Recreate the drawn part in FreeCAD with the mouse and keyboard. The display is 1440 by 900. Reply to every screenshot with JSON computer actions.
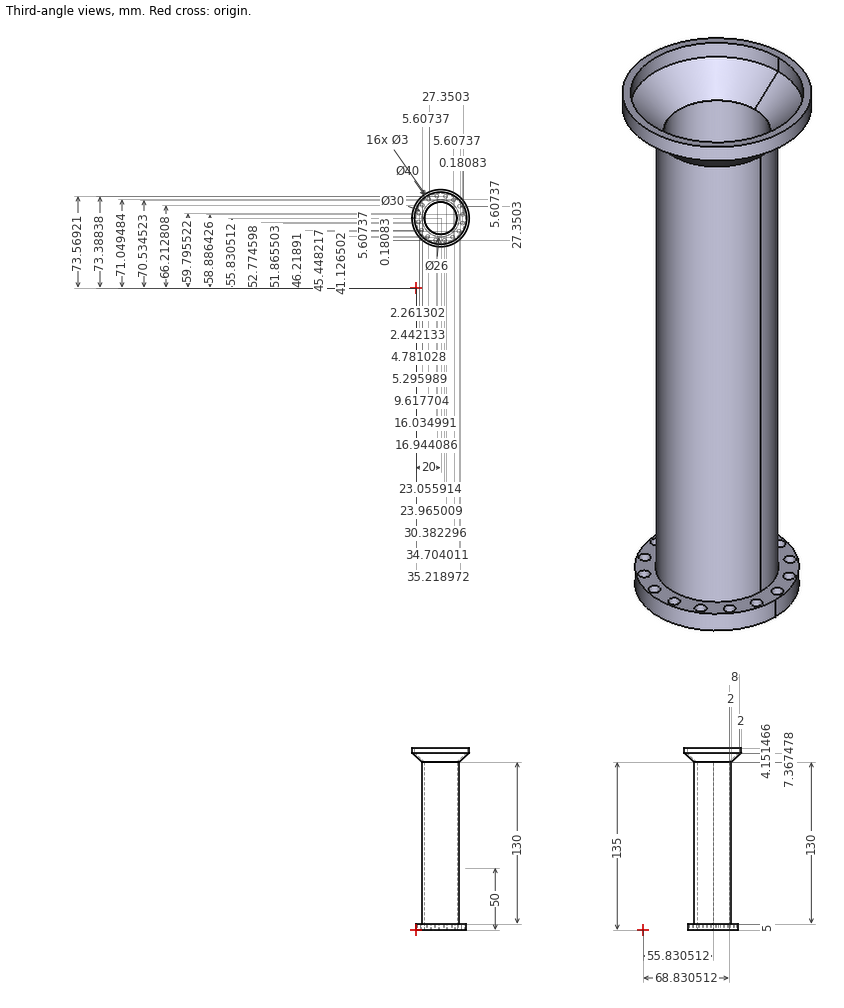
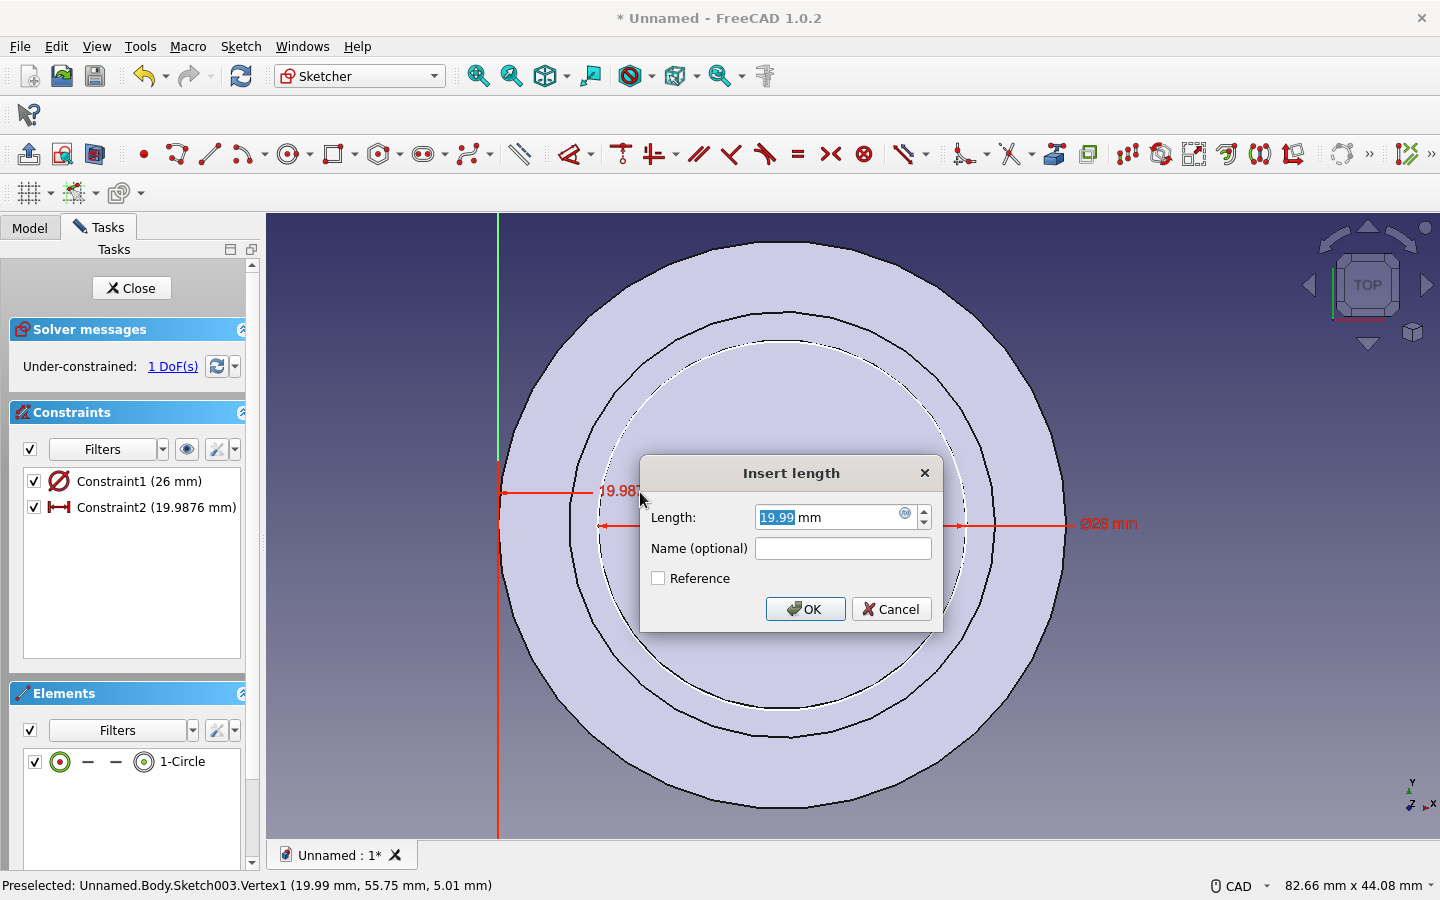
{"action": "type", "text": "20"}
{"action": "key", "text": "Return"}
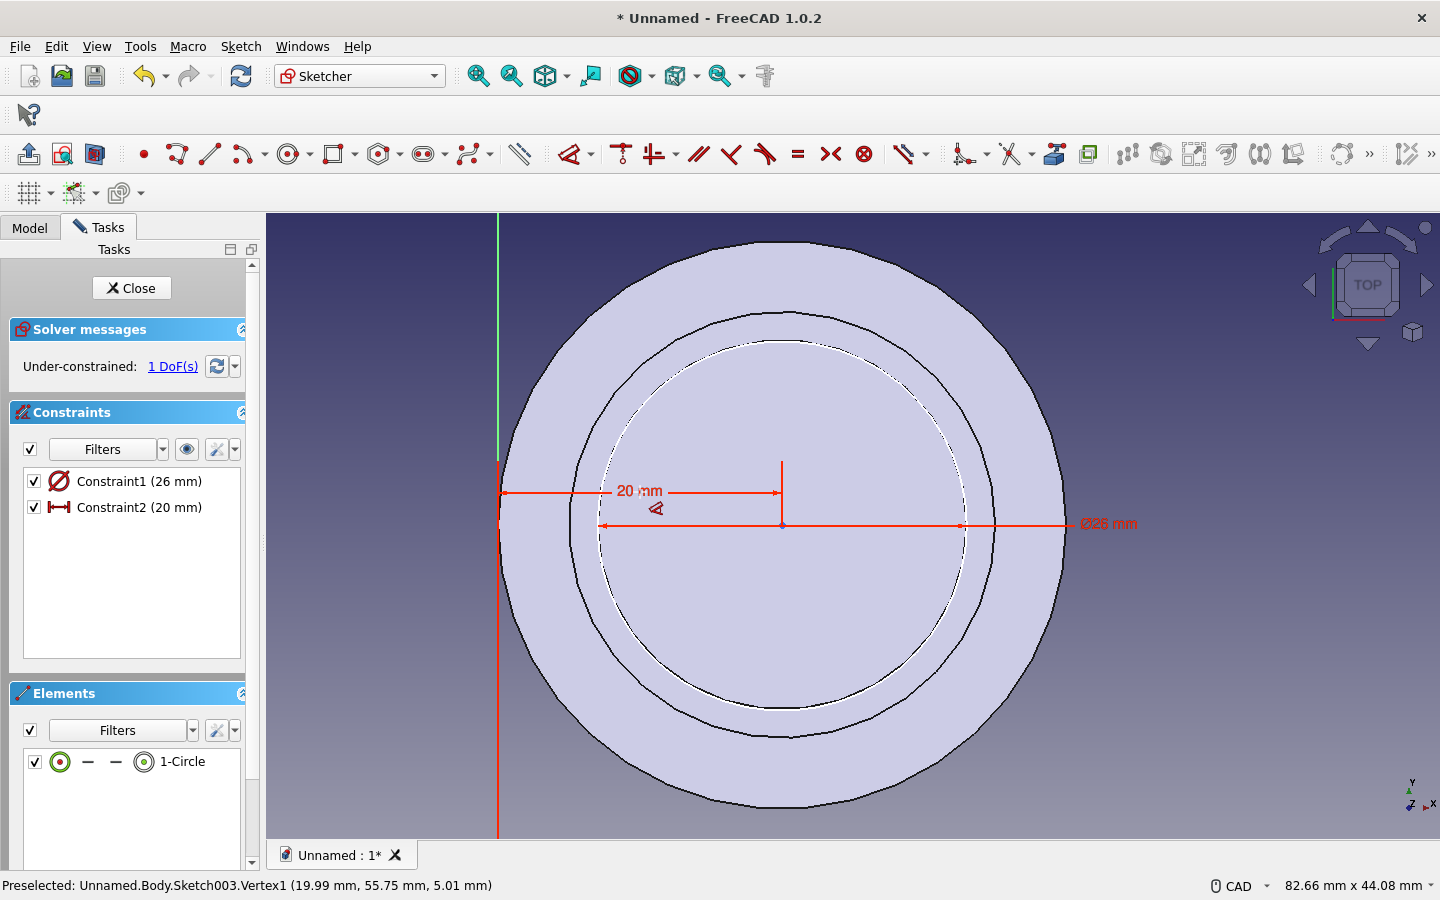
{"action": "left_click", "coordinate": [782, 526]}
{"action": "left_click", "coordinate": [464, 668]}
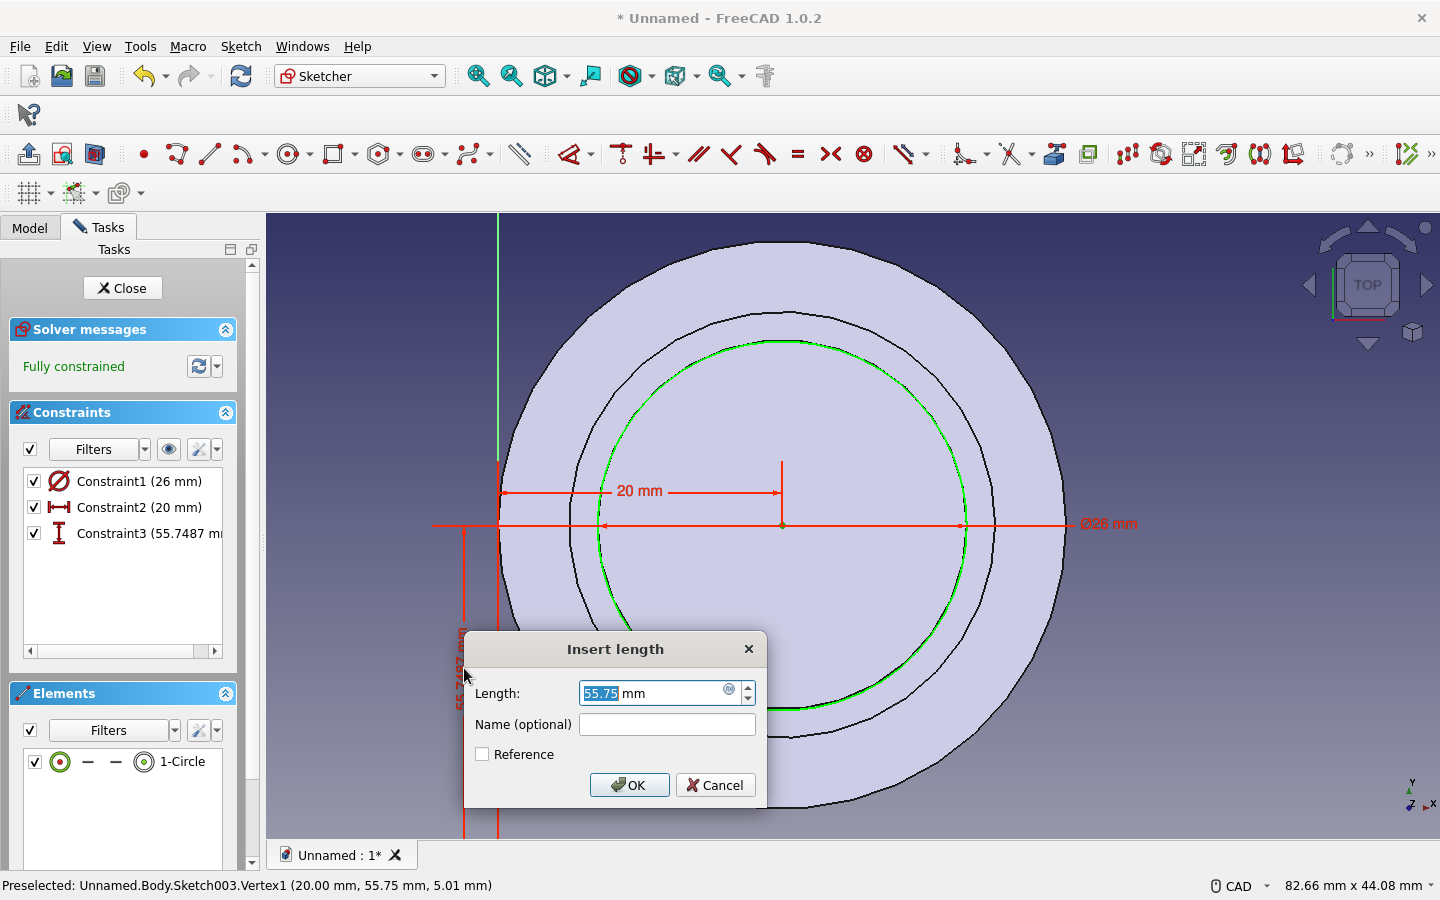
{"action": "type", "text": "55.830512"}
{"action": "key", "text": "Return"}
{"action": "key", "text": "Escape"}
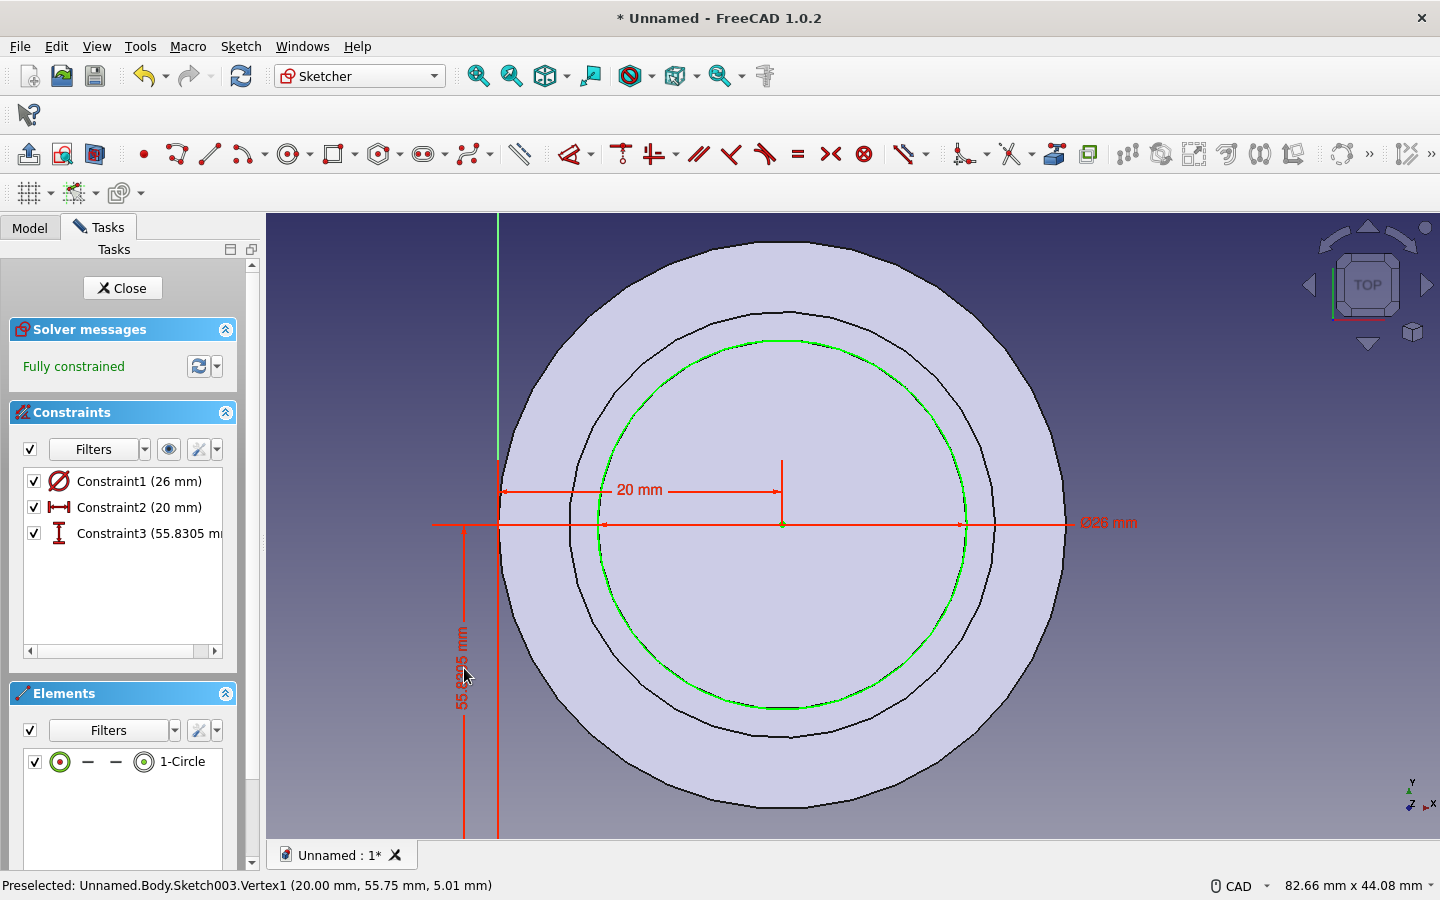
{"action": "left_click", "coordinate": [123, 288]}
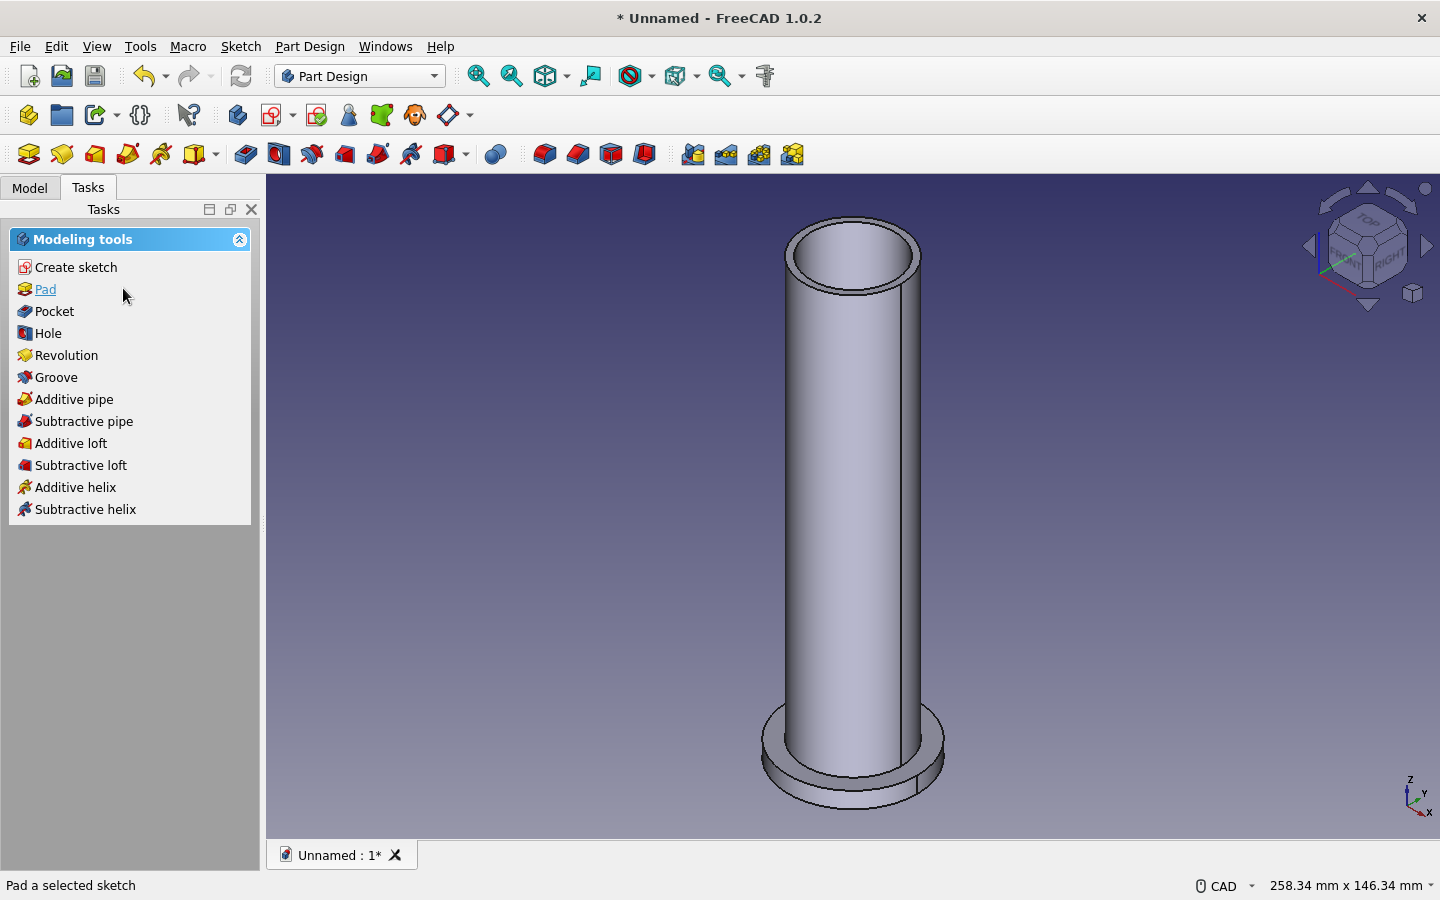
{"action": "left_click", "coordinate": [246, 154]}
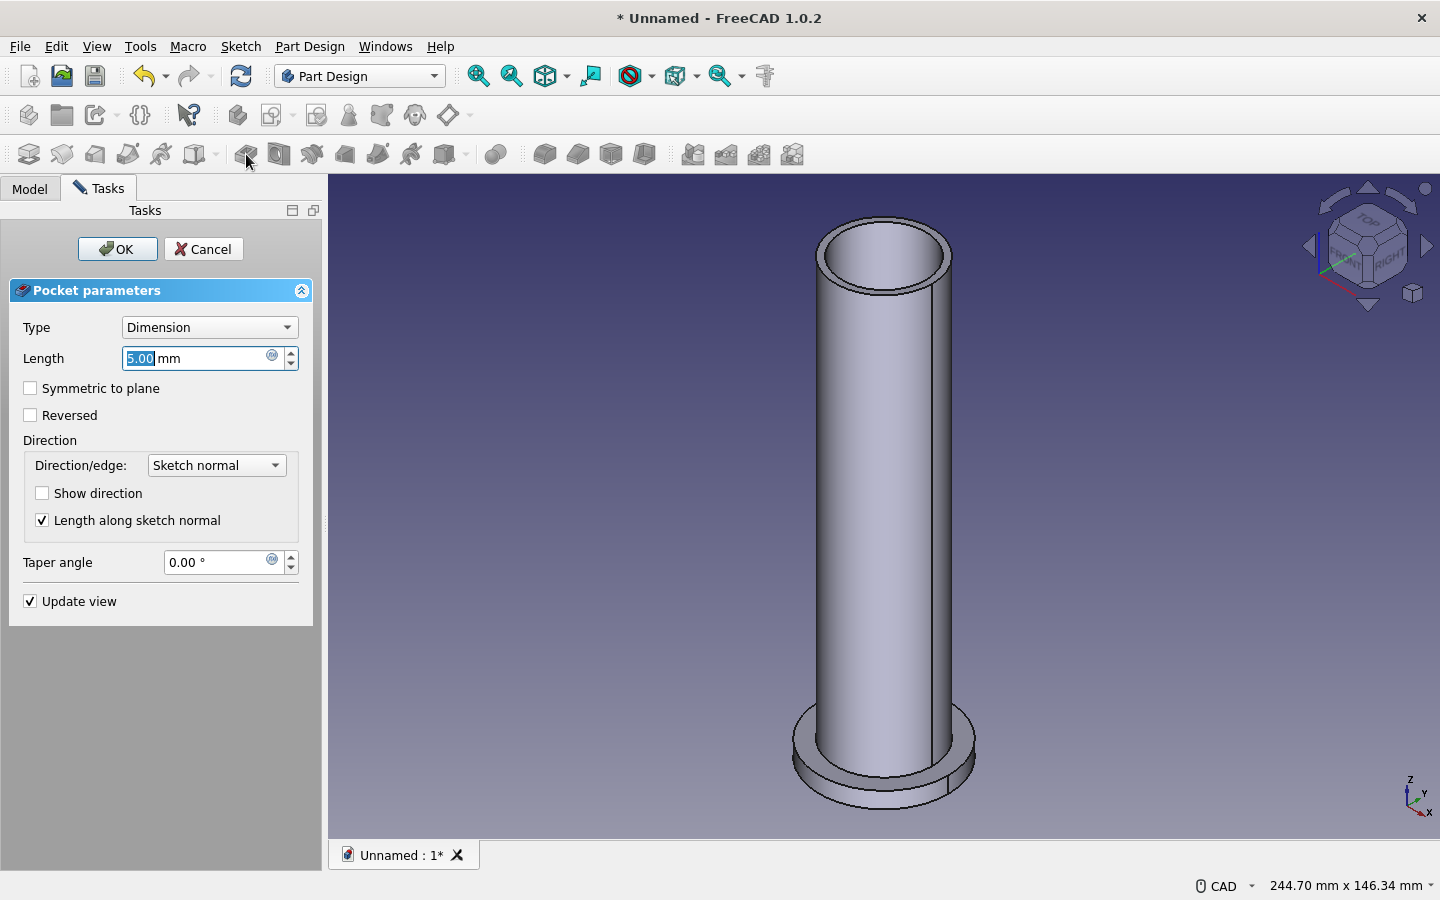
{"action": "left_click", "coordinate": [210, 328]}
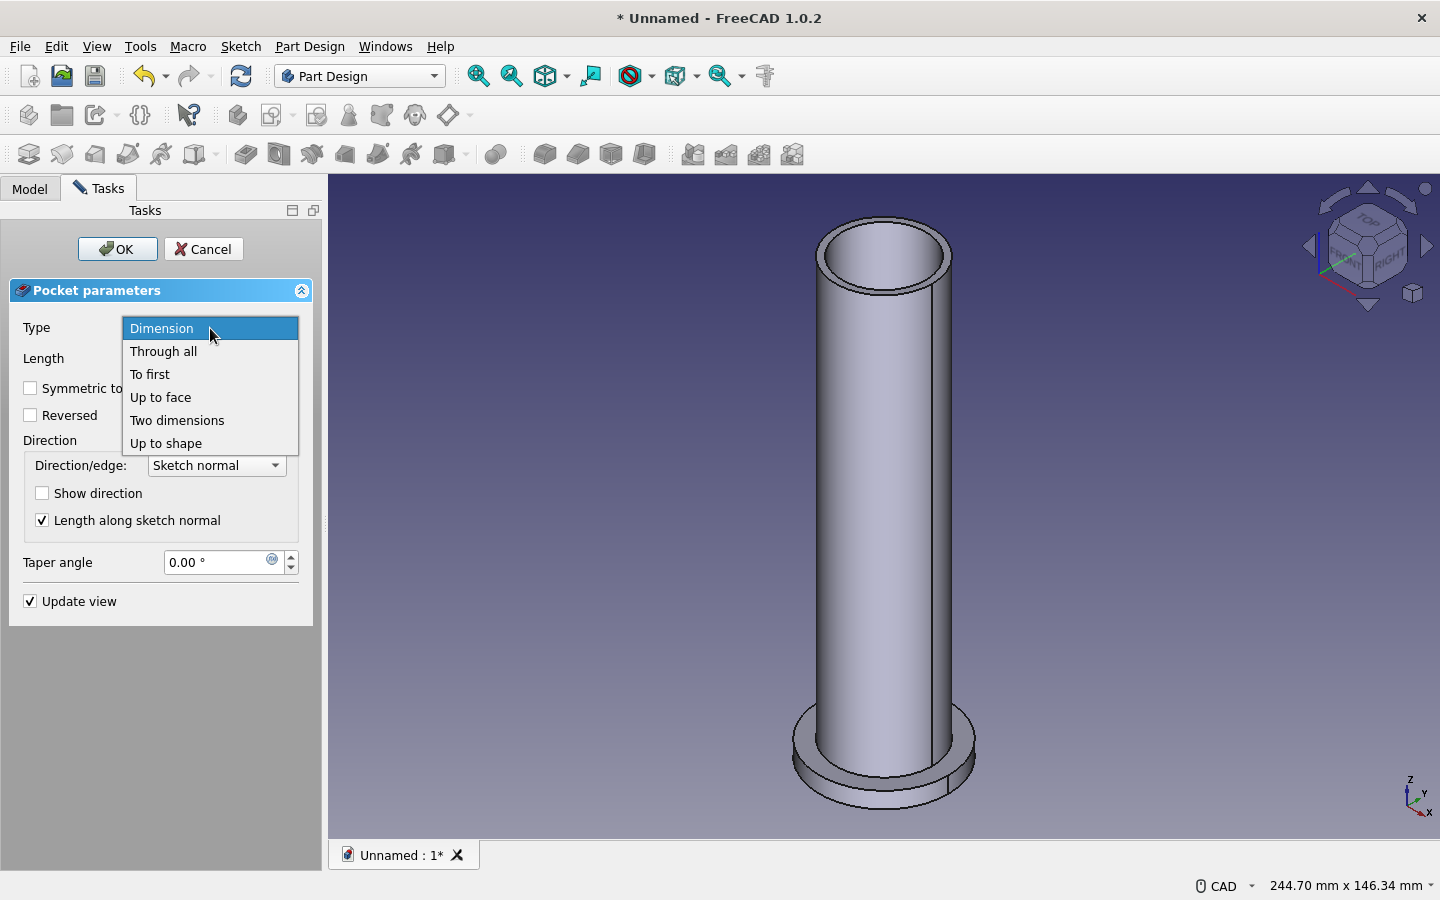
{"action": "left_click", "coordinate": [208, 352]}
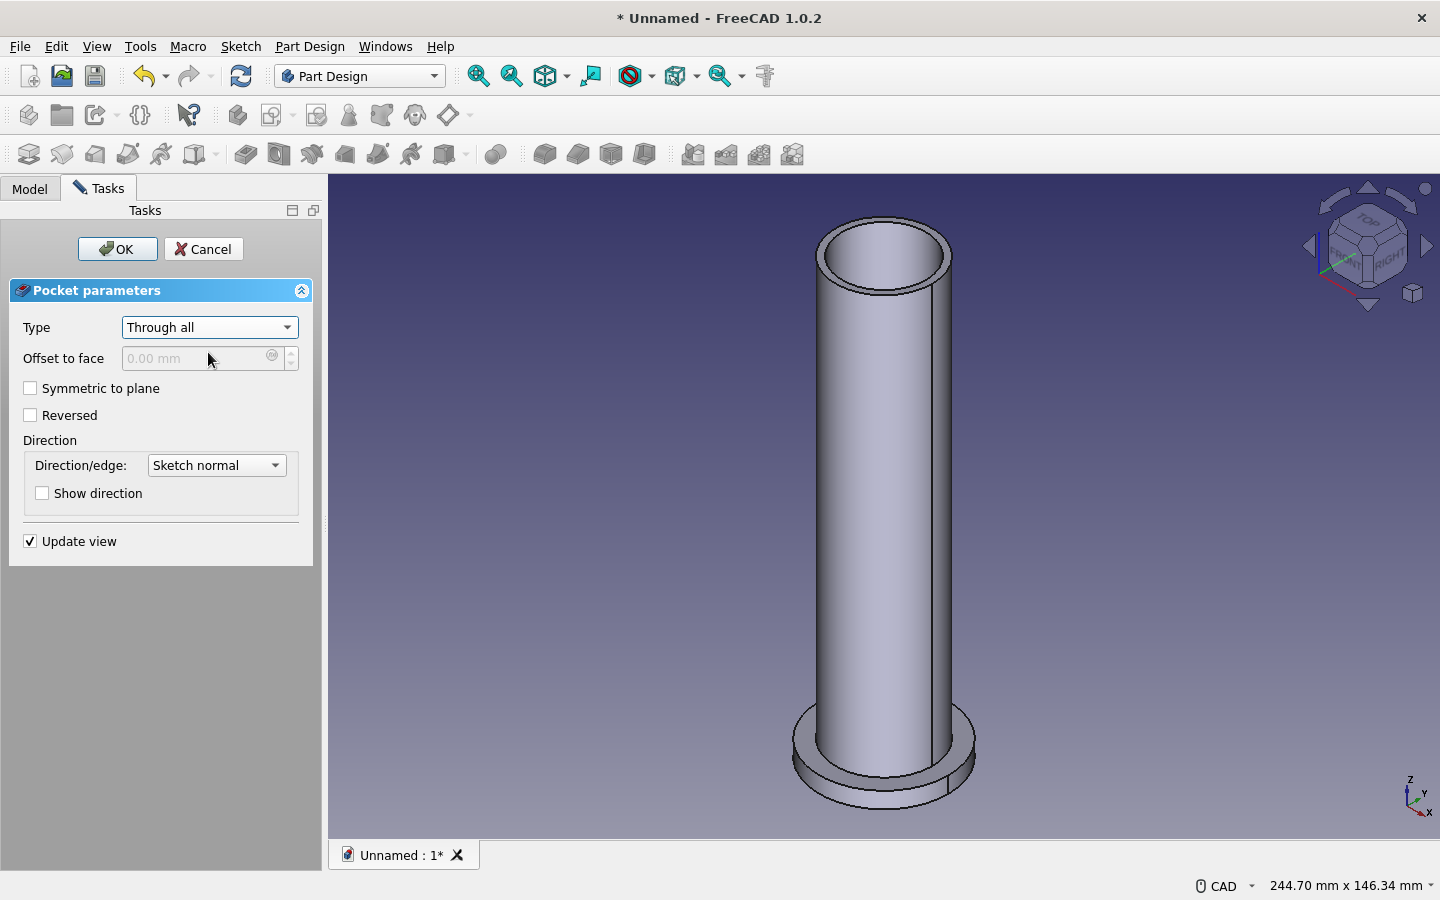
{"action": "left_click", "coordinate": [118, 249]}